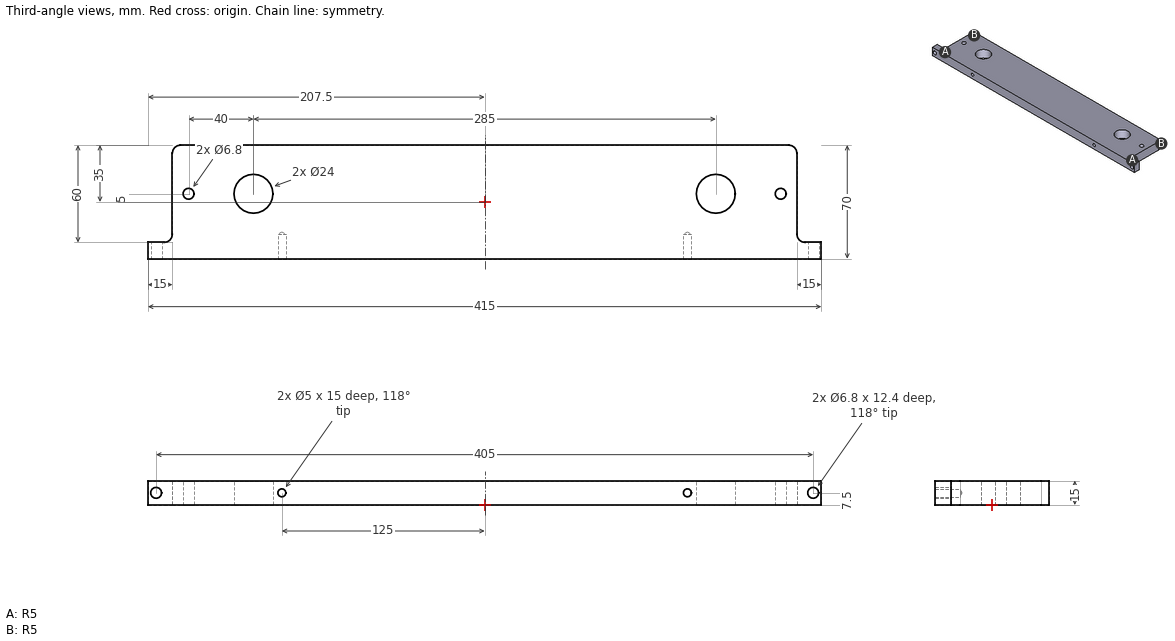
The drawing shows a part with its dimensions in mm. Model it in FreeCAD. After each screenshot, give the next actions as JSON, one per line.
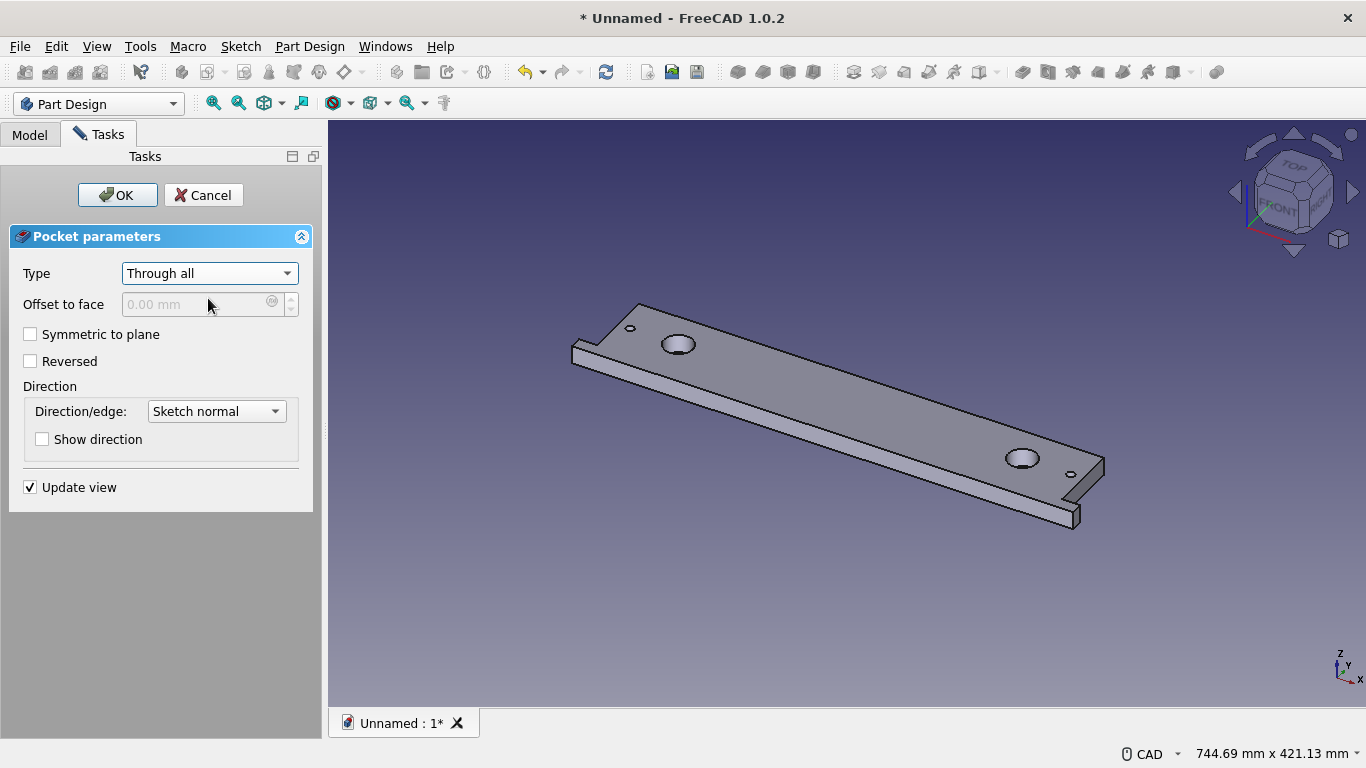
{"action": "left_click", "coordinate": [118, 195]}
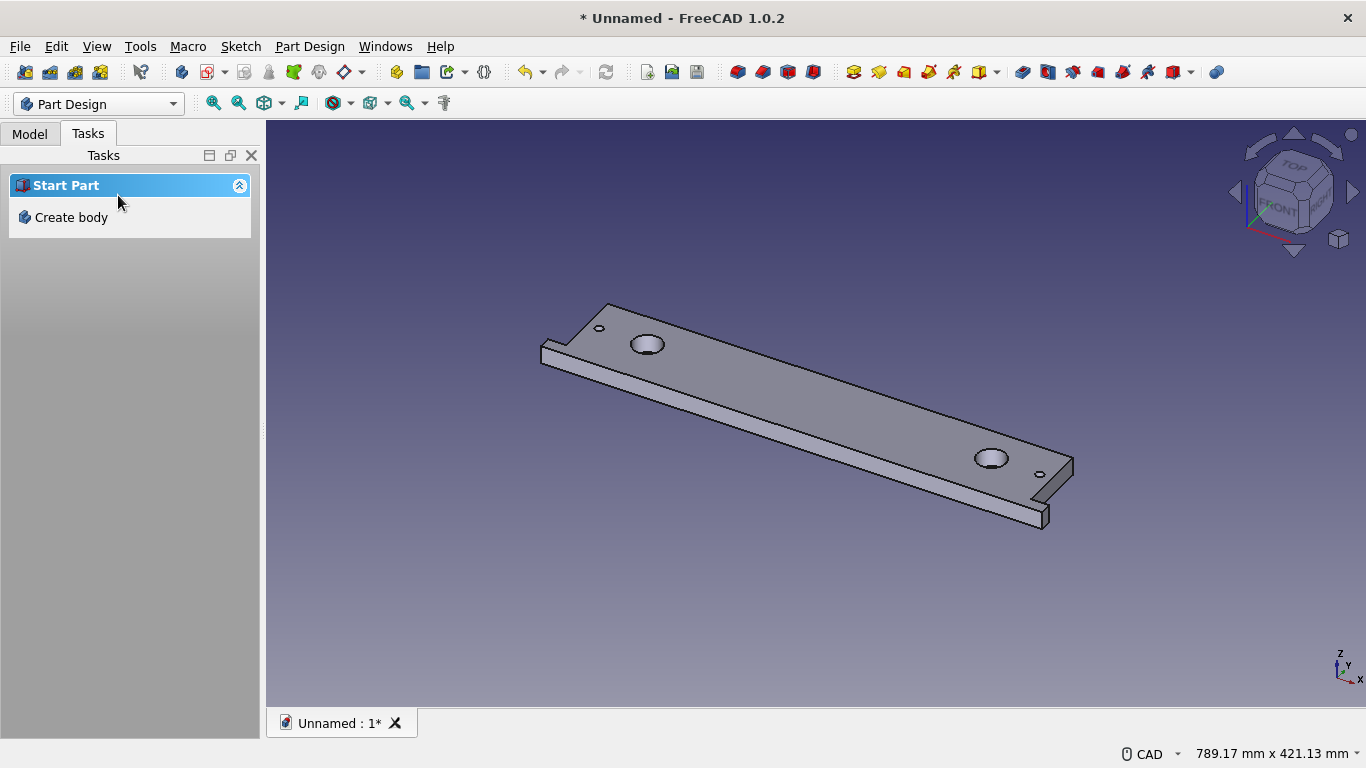
{"action": "key", "text": "0"}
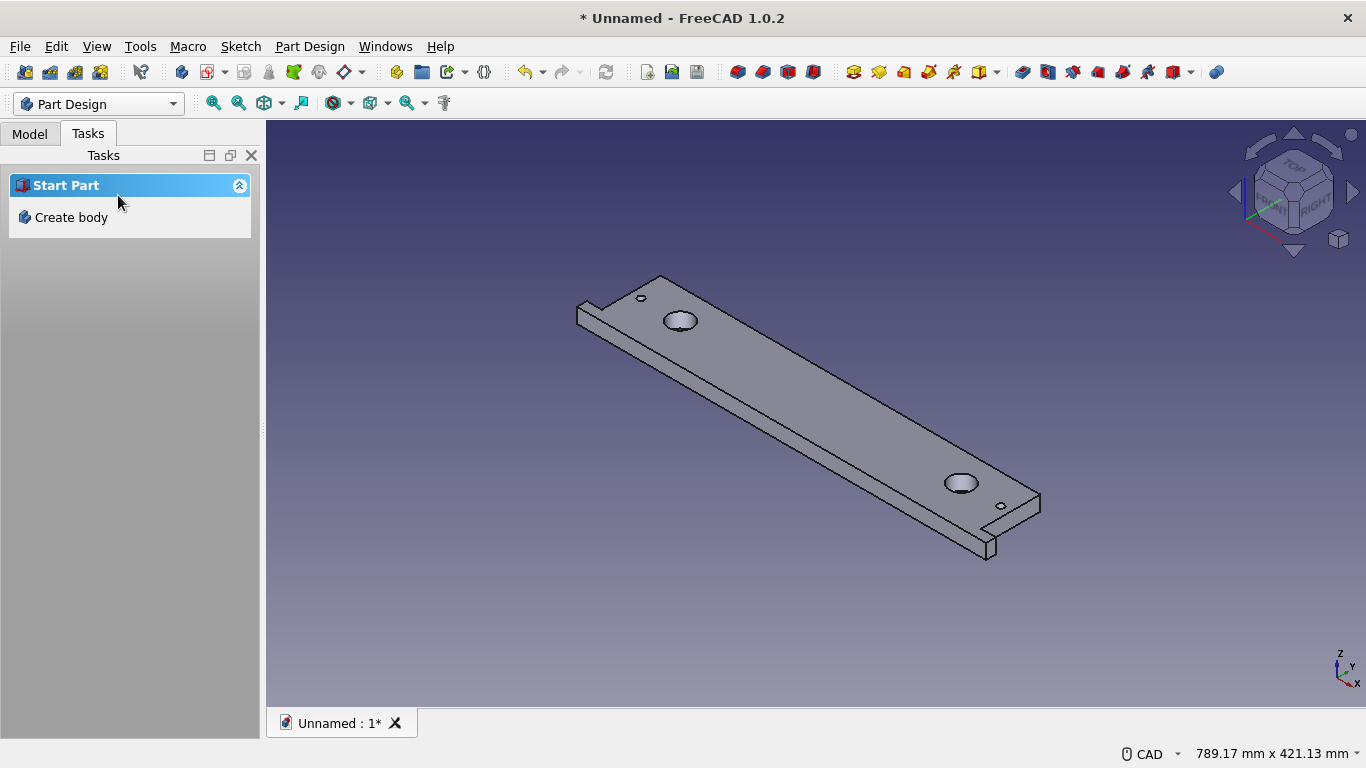
{"action": "key", "text": "1"}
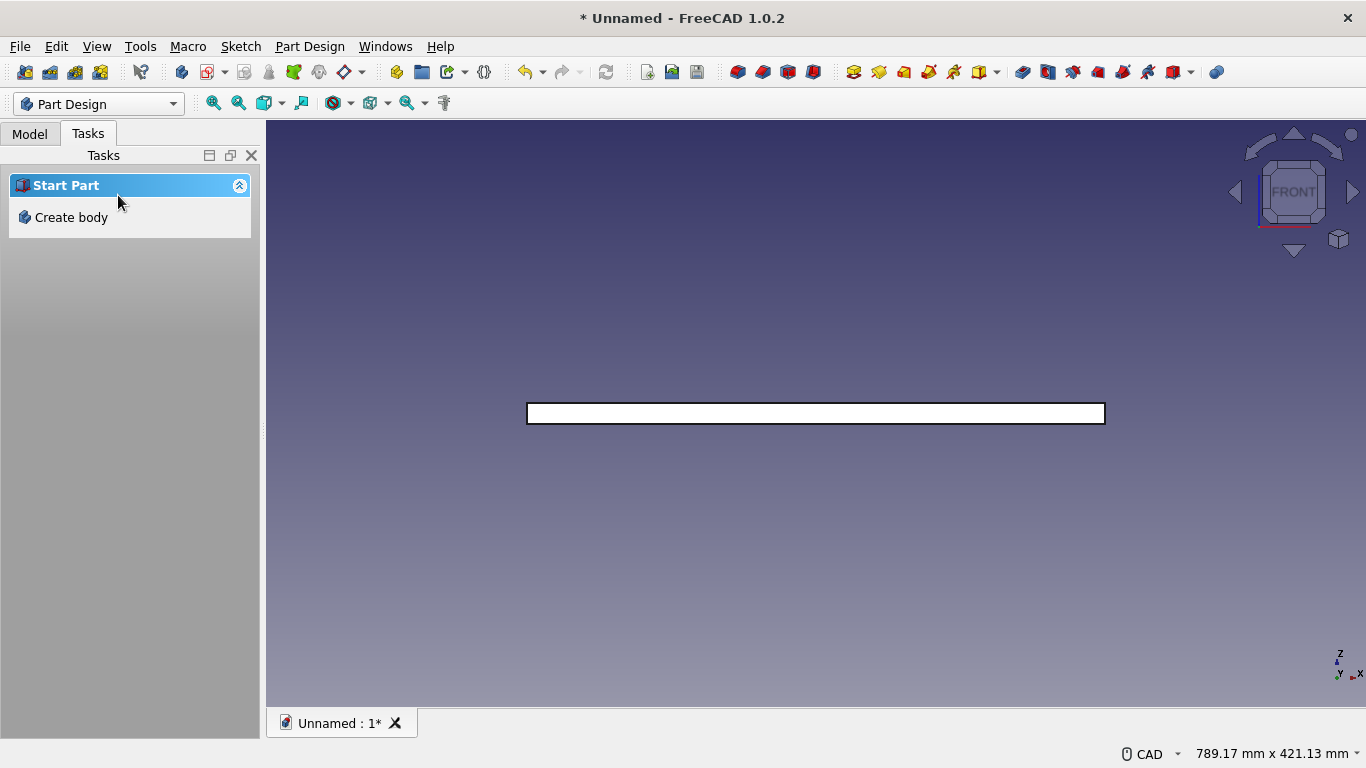
{"action": "left_click", "coordinate": [1064, 412]}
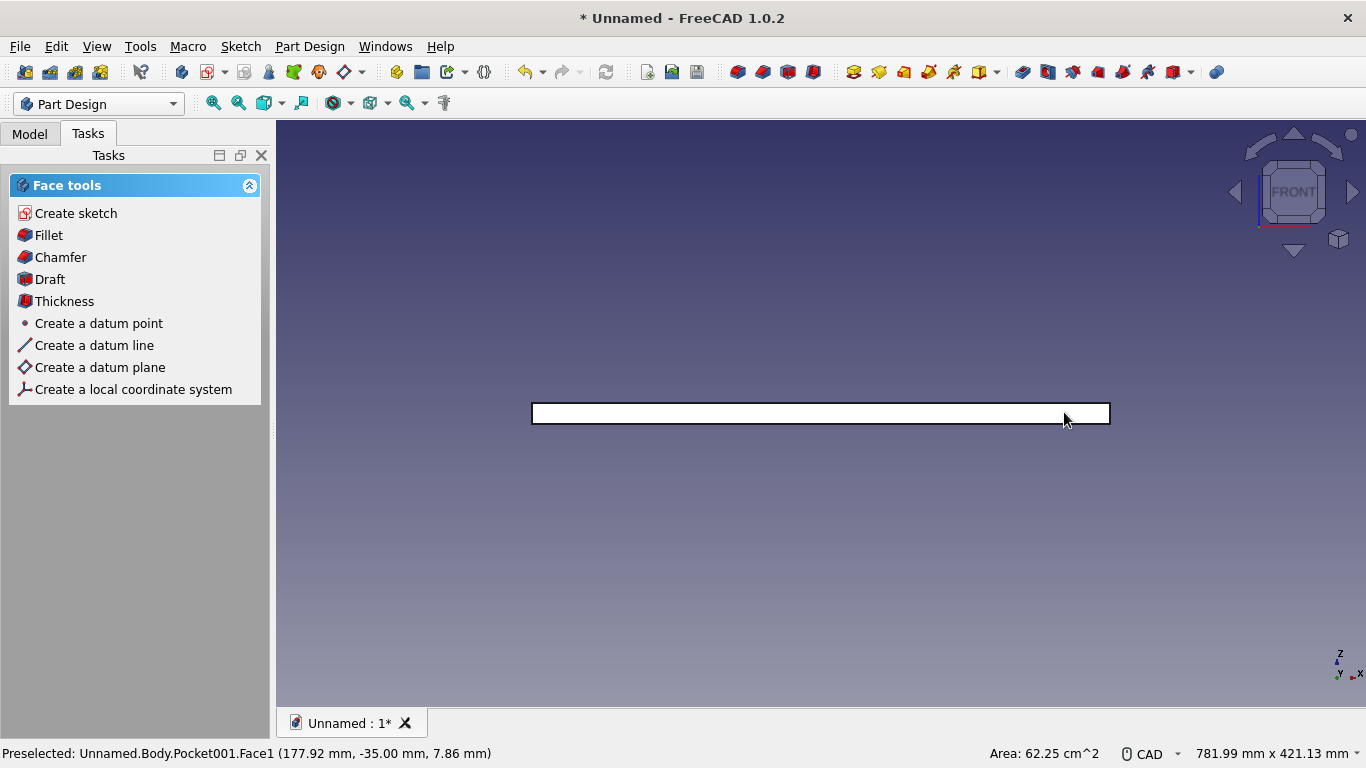
{"action": "left_click", "coordinate": [206, 72]}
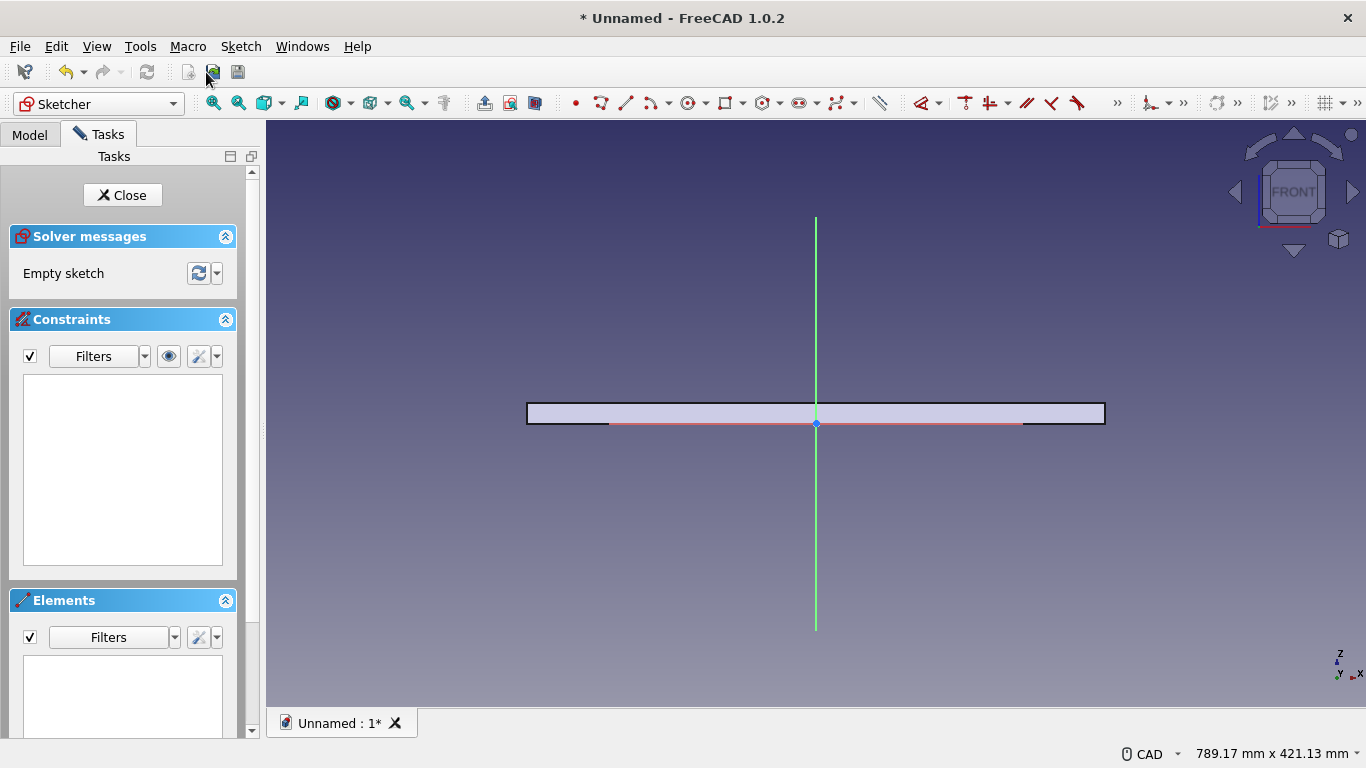
{"action": "key", "text": "g c"}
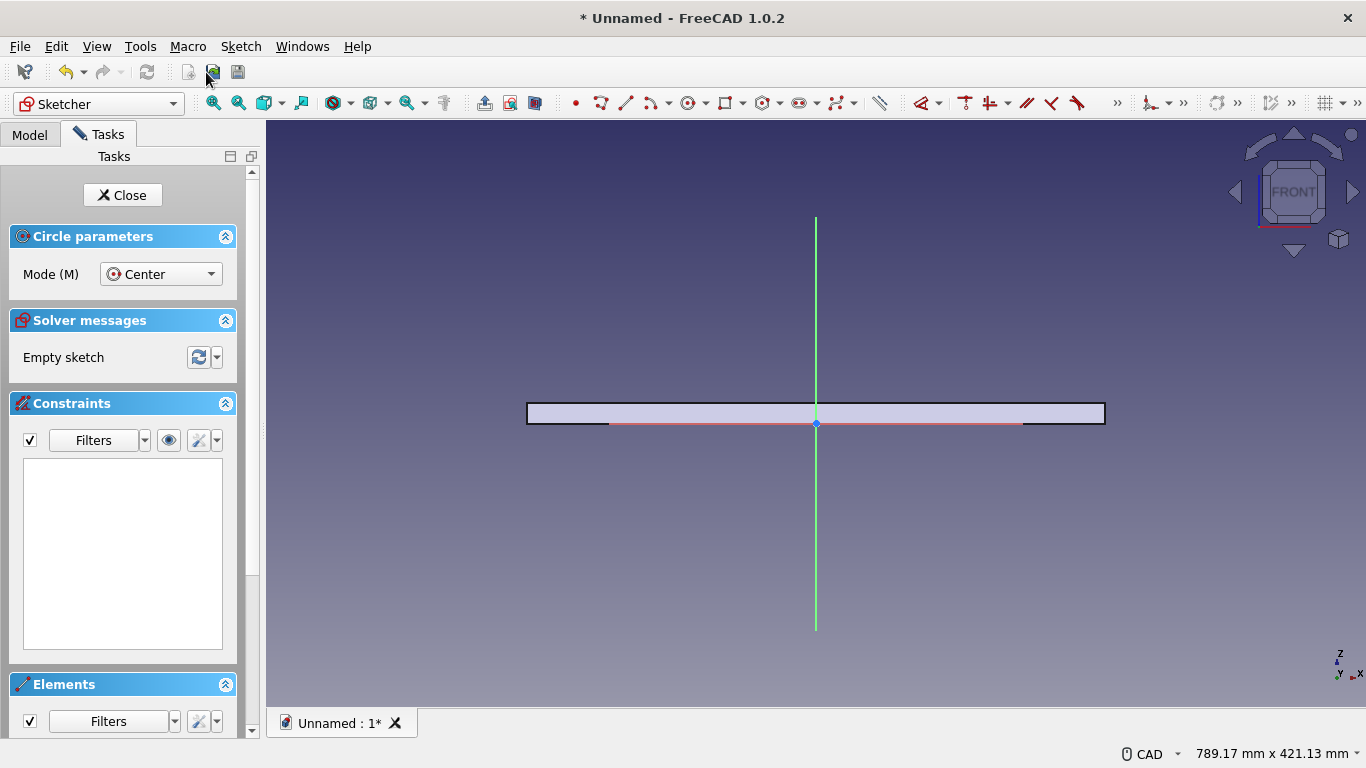
{"action": "scroll", "coordinate": [1098, 413], "scroll_direction": "up", "scroll_amount": 8}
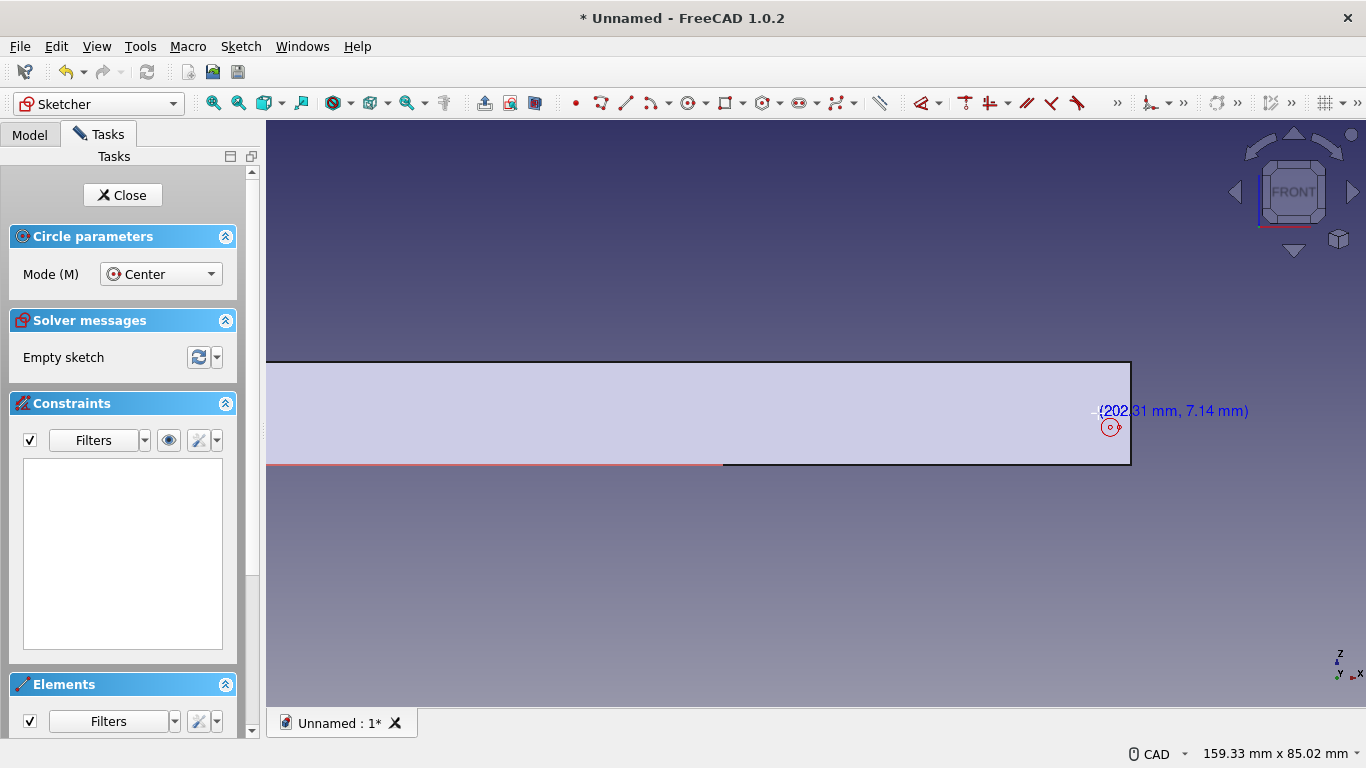
{"action": "scroll", "coordinate": [1091, 409], "scroll_direction": "down", "scroll_amount": 7}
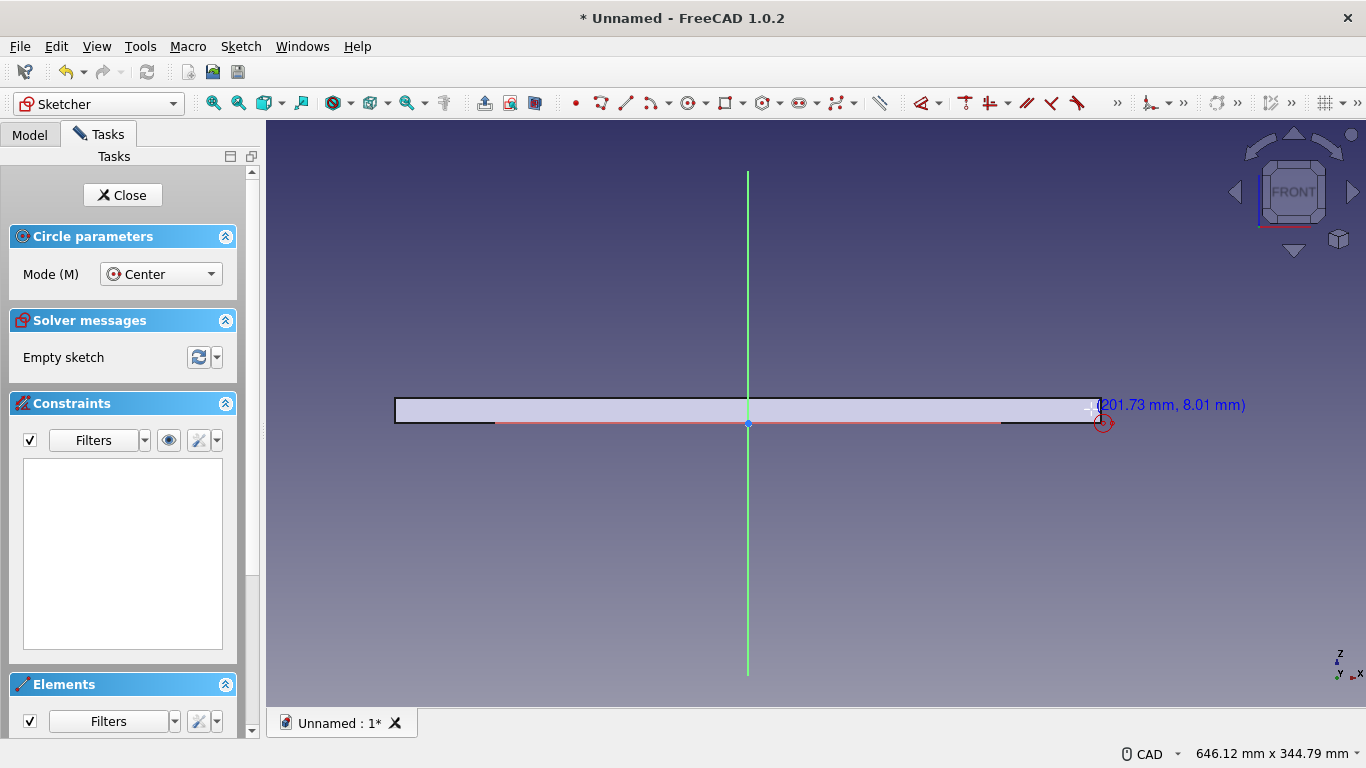
{"action": "scroll", "coordinate": [1093, 410], "scroll_direction": "up", "scroll_amount": 2}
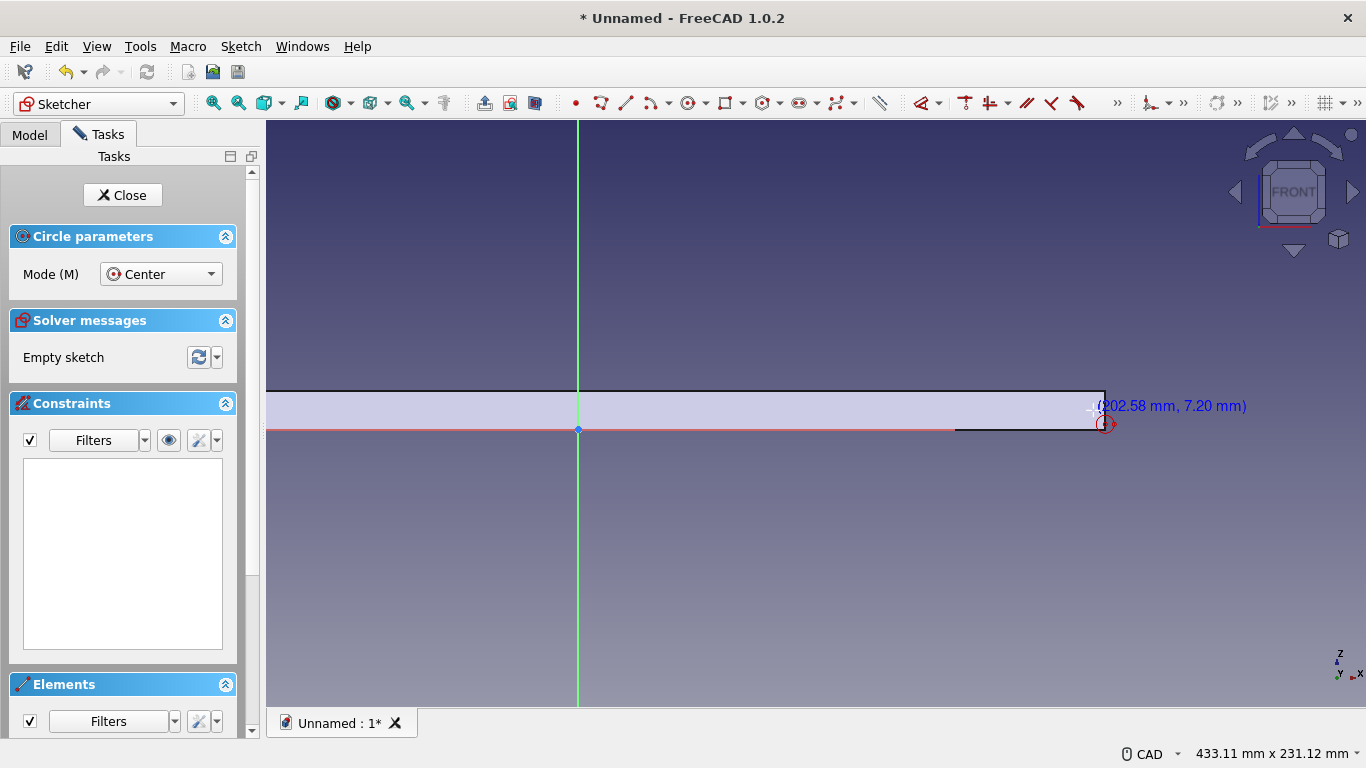
{"action": "left_click", "coordinate": [1092, 410]}
{"action": "mouse_move", "coordinate": [1099, 404]}